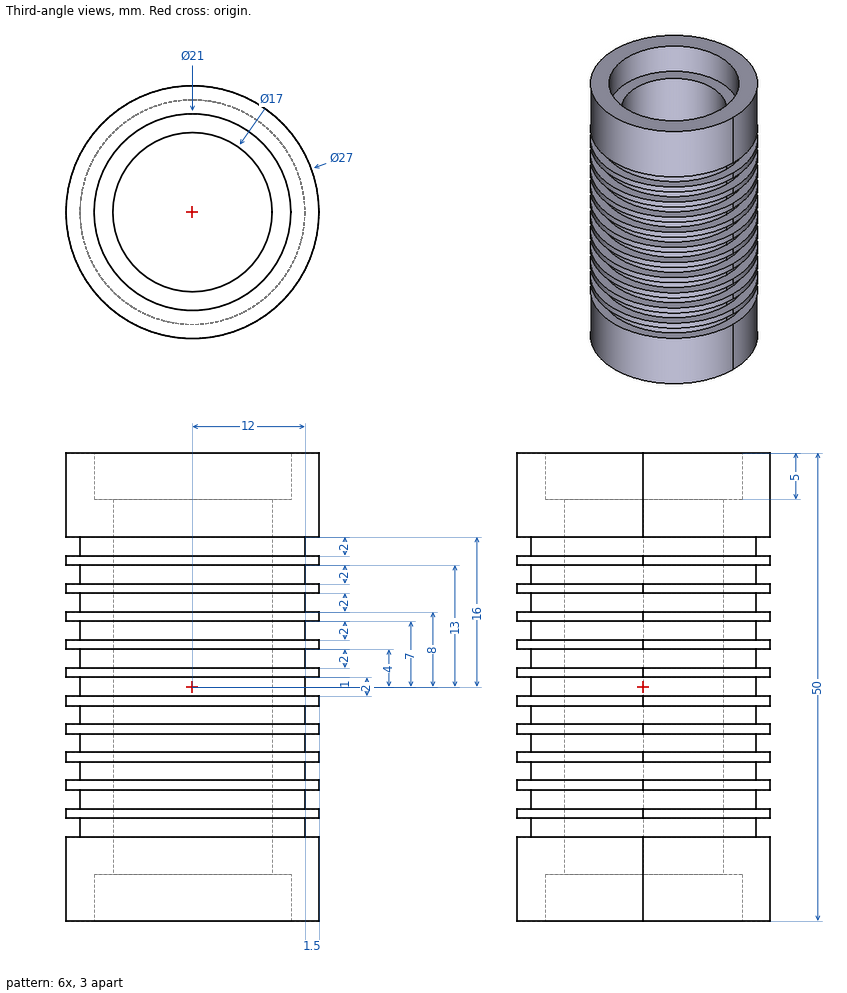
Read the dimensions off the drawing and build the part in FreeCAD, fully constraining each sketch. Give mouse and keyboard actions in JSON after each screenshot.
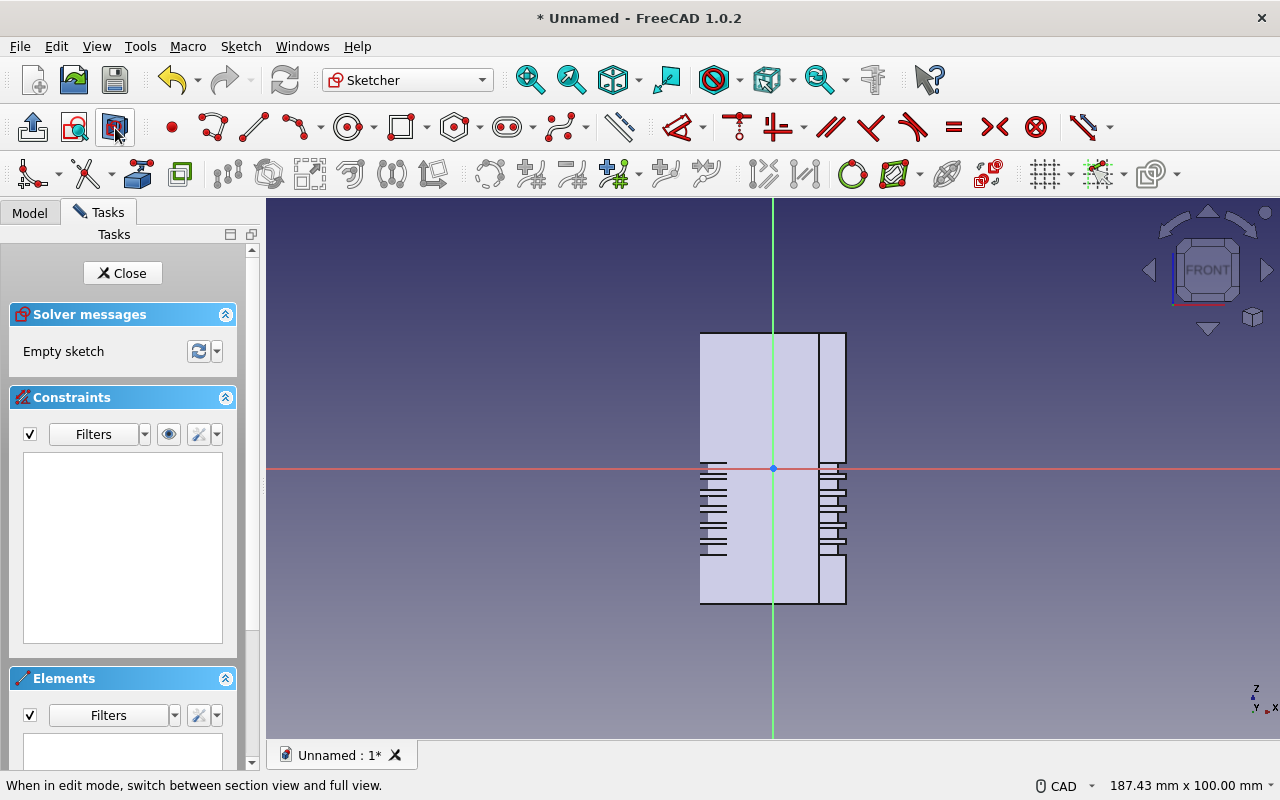
{"action": "scroll", "coordinate": [849, 451], "scroll_direction": "up", "scroll_amount": 15}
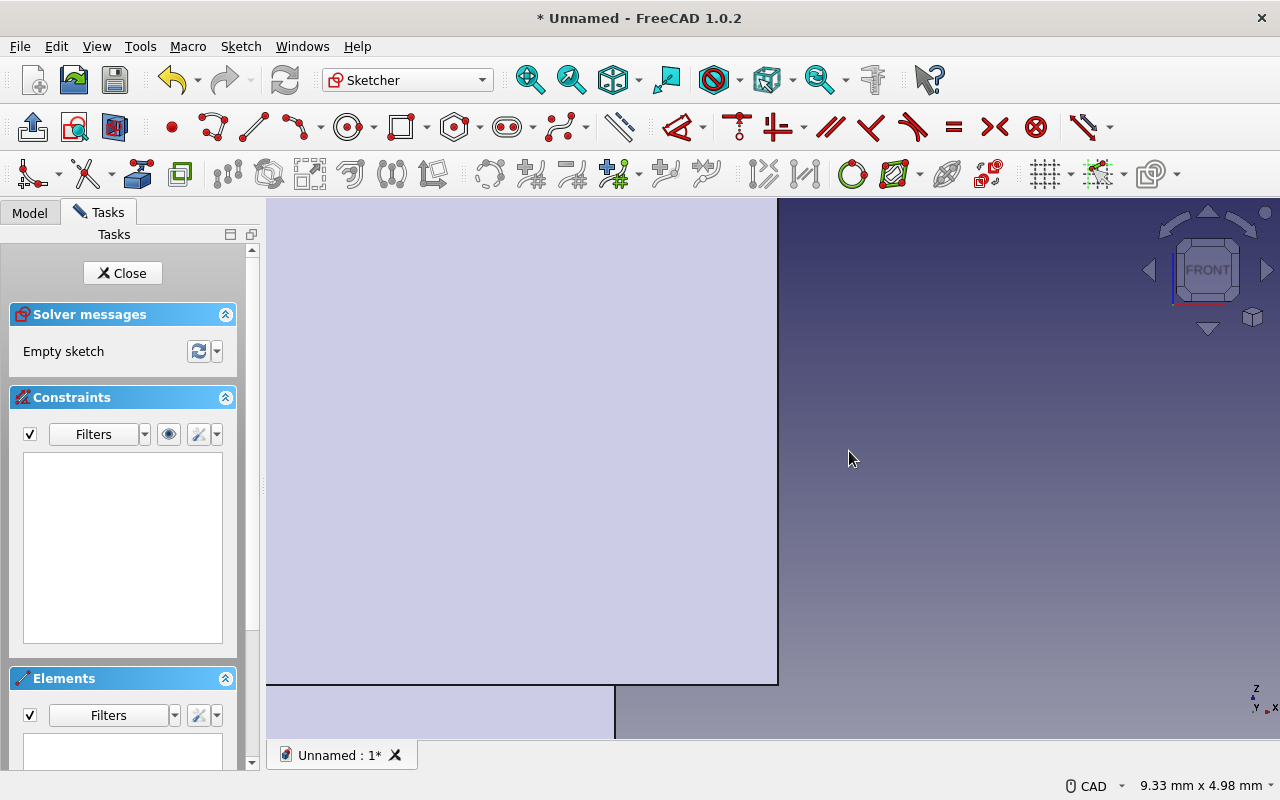
{"action": "scroll", "coordinate": [682, 466], "scroll_direction": "up", "scroll_amount": 2}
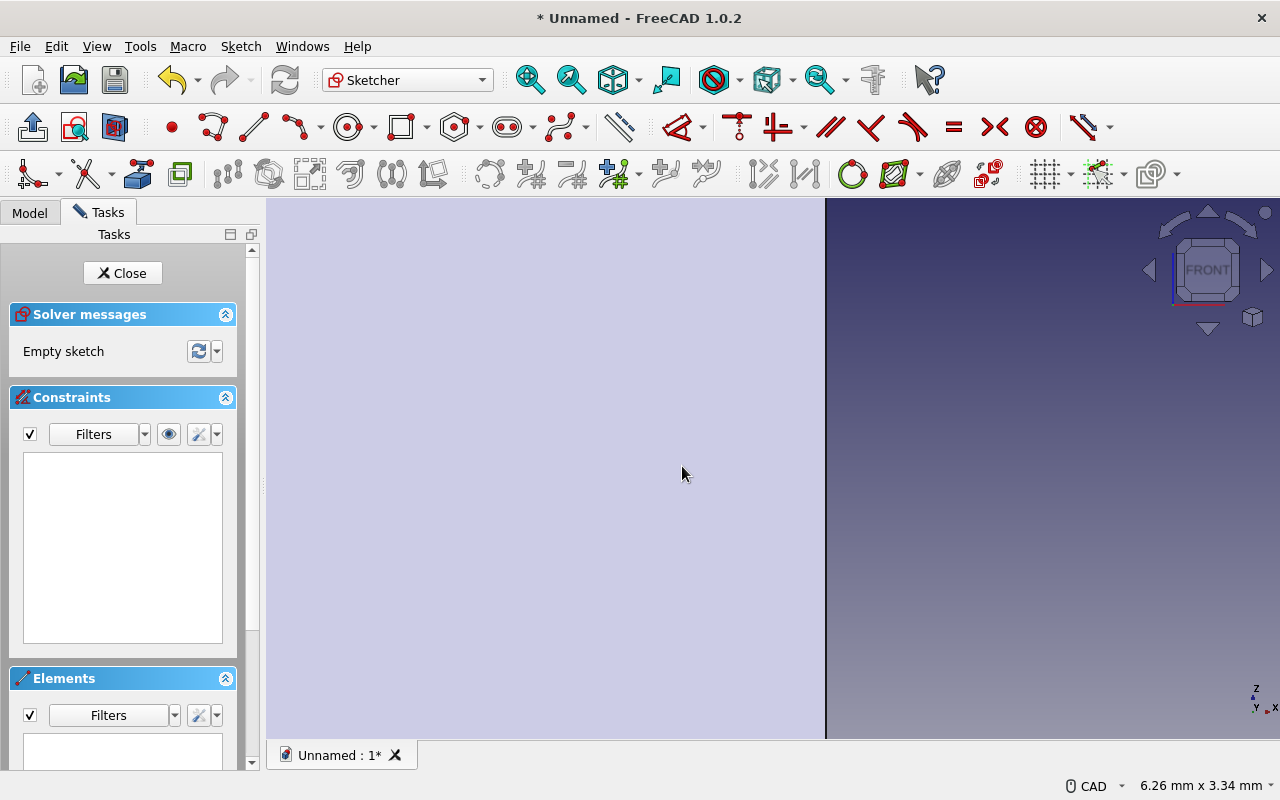
{"action": "left_click", "coordinate": [400, 128]}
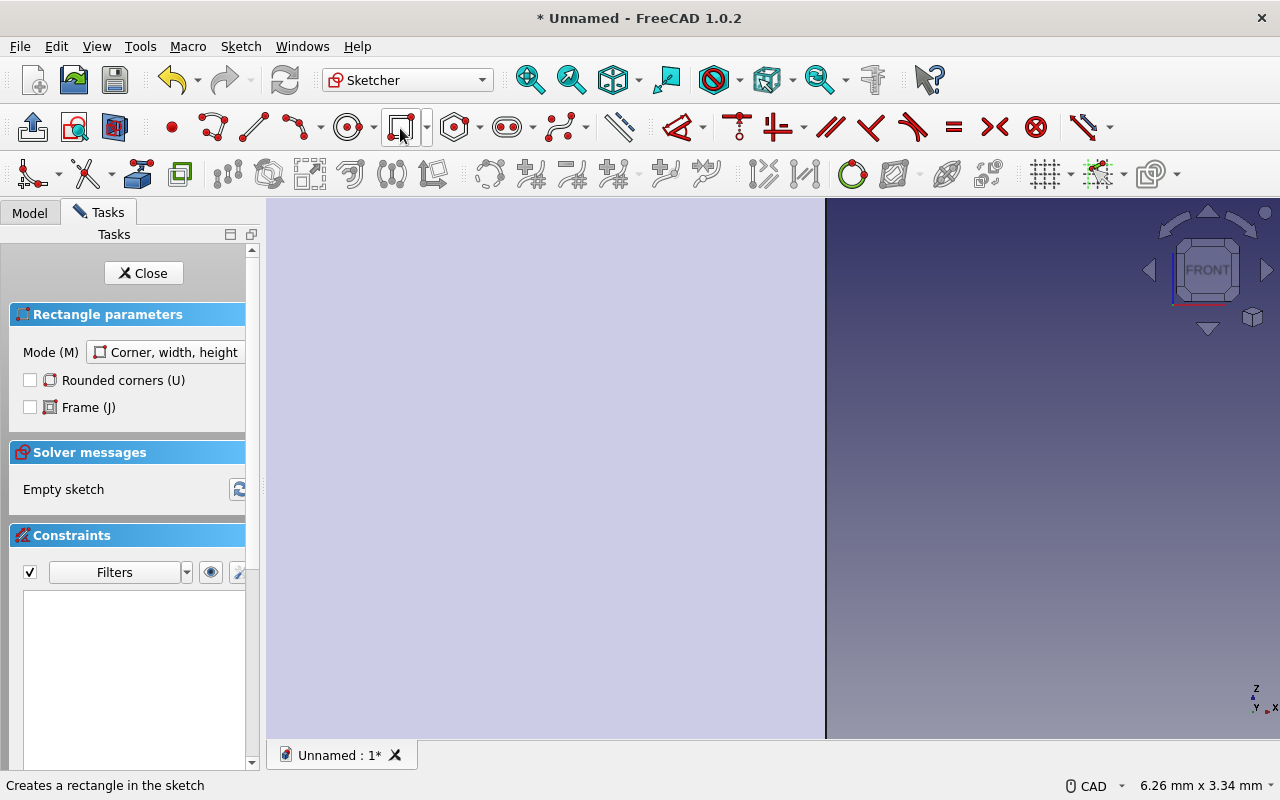
{"action": "left_click", "coordinate": [583, 306]}
{"action": "mouse_move", "coordinate": [826, 630]}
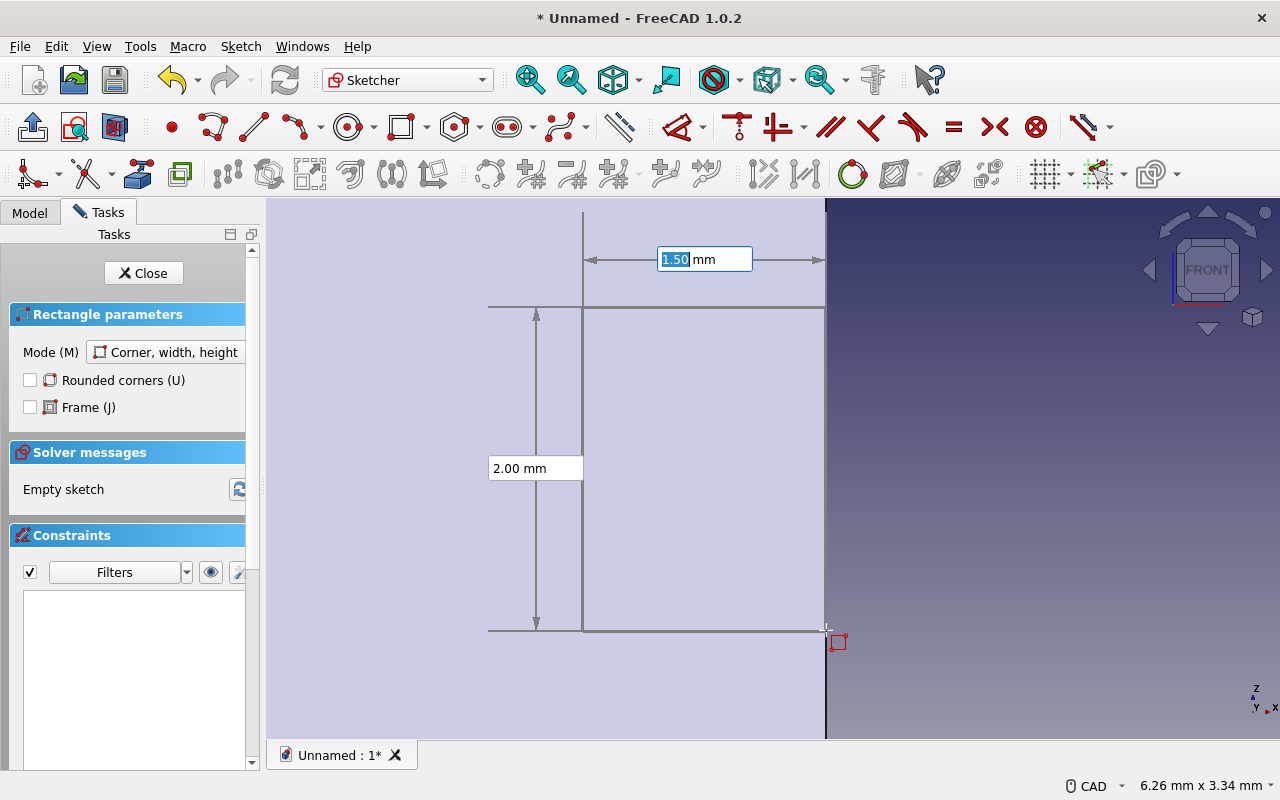
{"action": "type", "text": "1.5"}
{"action": "key", "text": "Tab"}
{"action": "type", "text": "2"}
{"action": "key", "text": "Return"}
{"action": "key", "text": "Escape"}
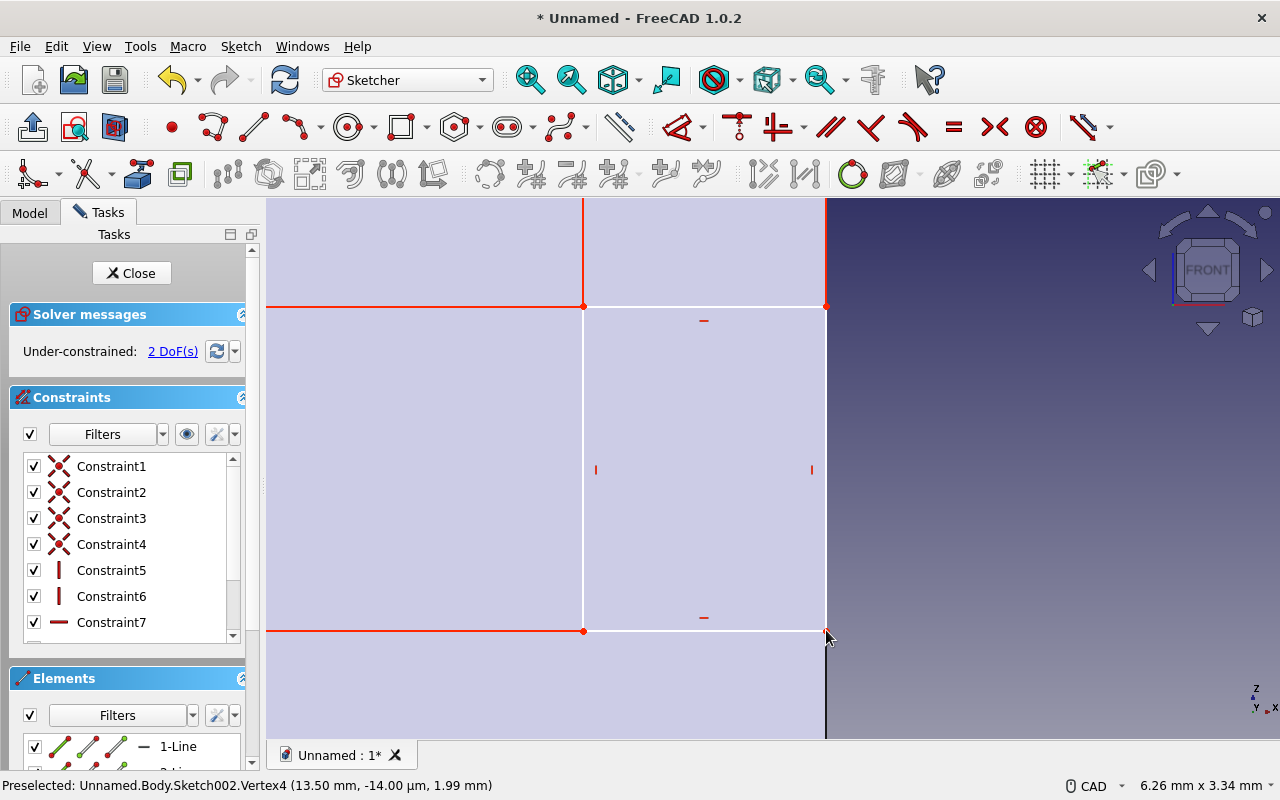
{"action": "left_click", "coordinate": [676, 128]}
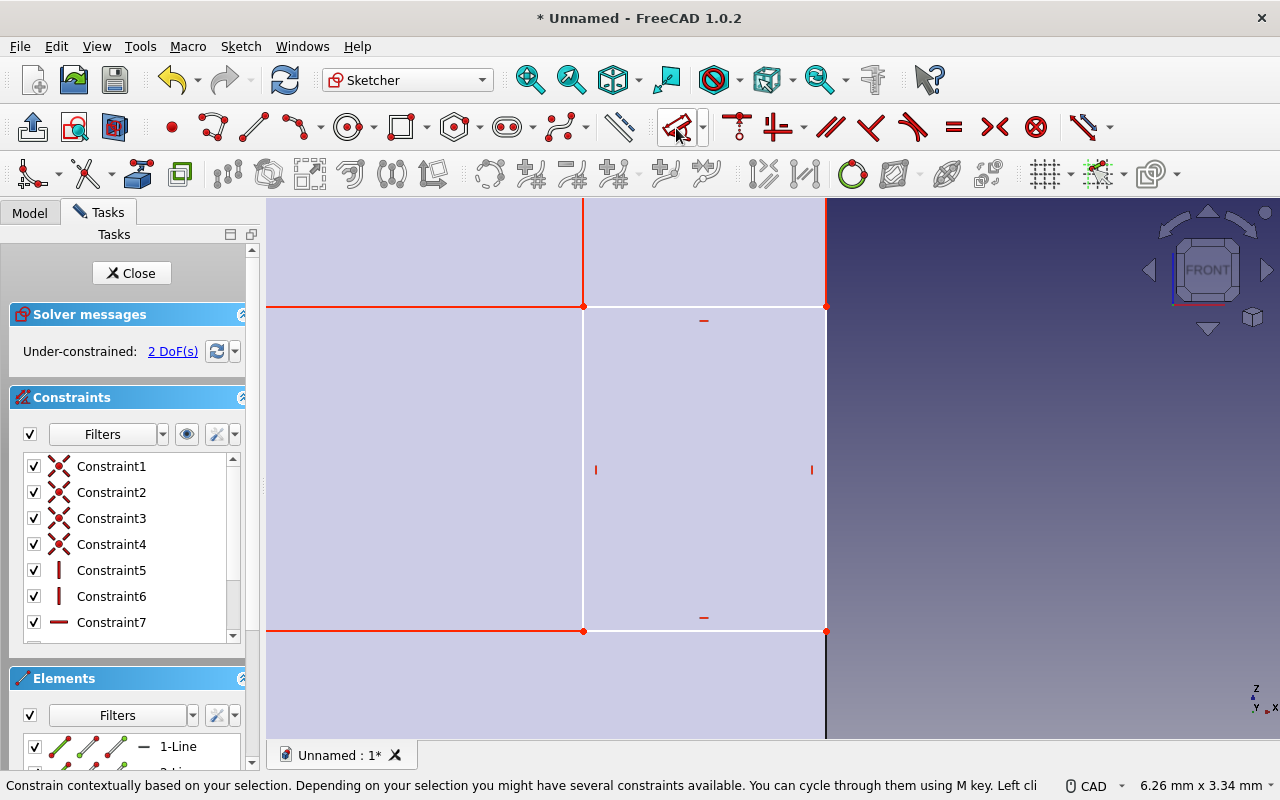
{"action": "left_click", "coordinate": [583, 307]}
{"action": "left_click", "coordinate": [617, 509]}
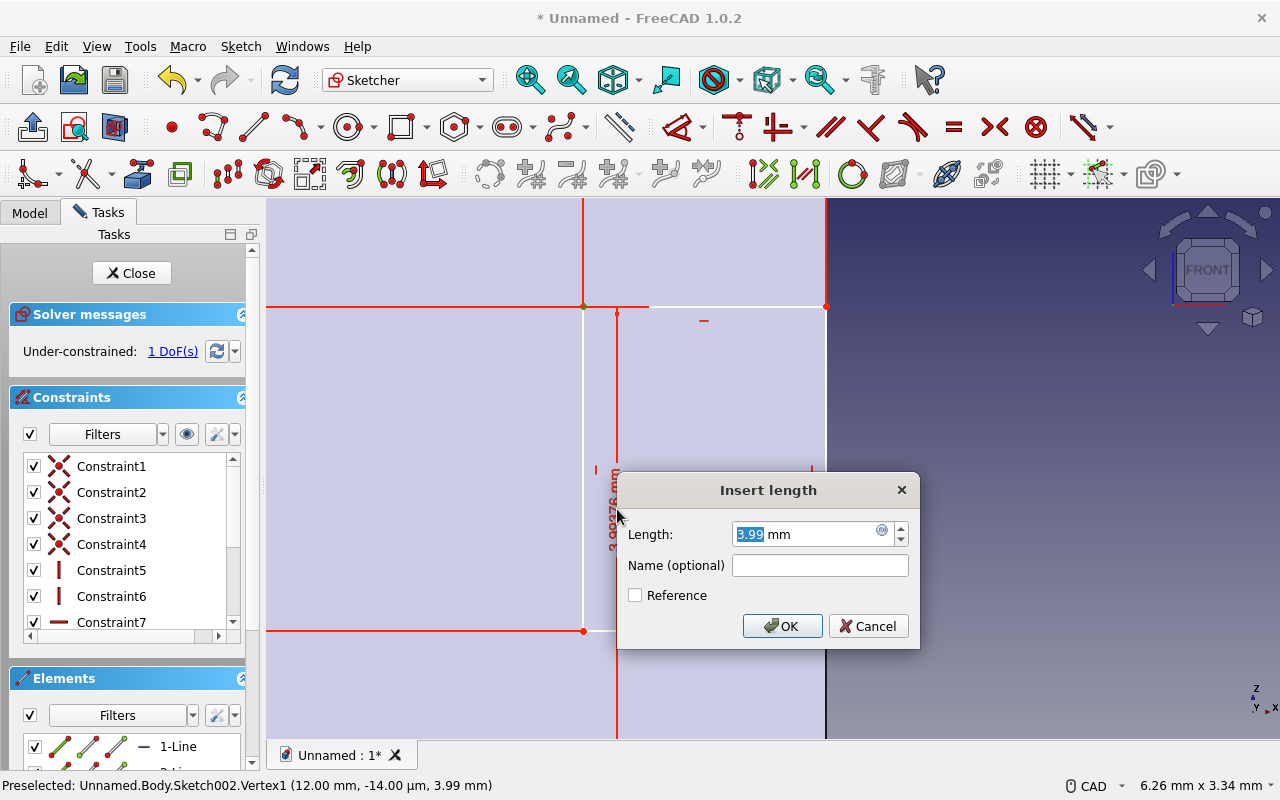
{"action": "type", "text": "4"}
{"action": "key", "text": "Return"}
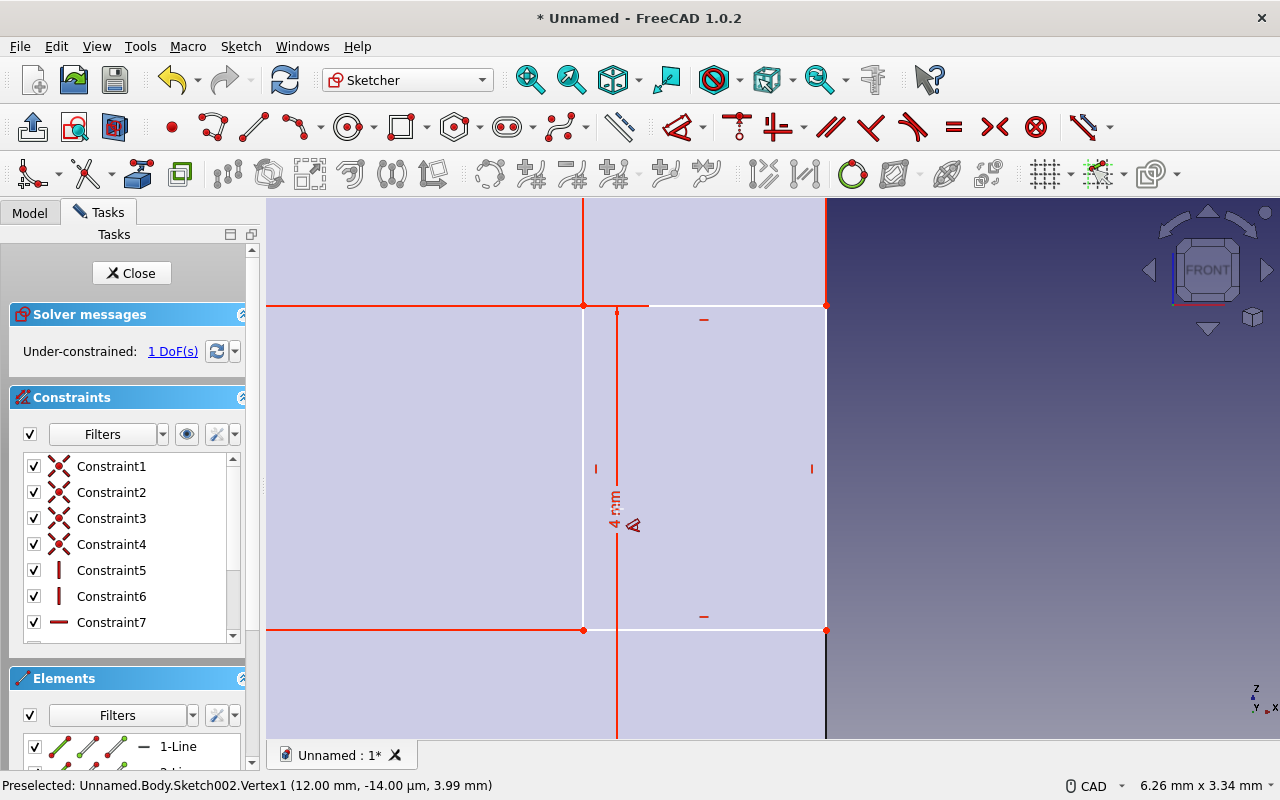
{"action": "left_click", "coordinate": [583, 306]}
{"action": "left_click", "coordinate": [438, 272]}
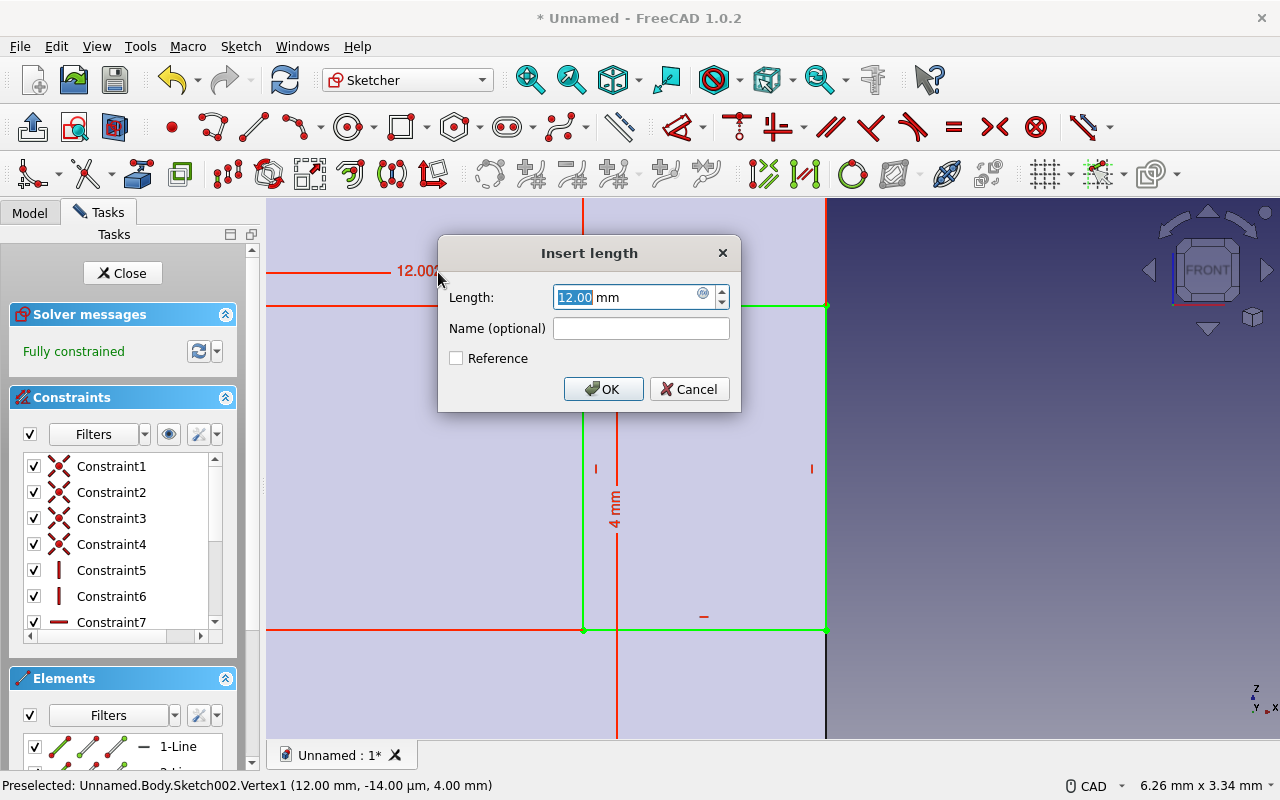
{"action": "type", "text": "12"}
{"action": "key", "text": "Return"}
{"action": "key", "text": "Escape"}